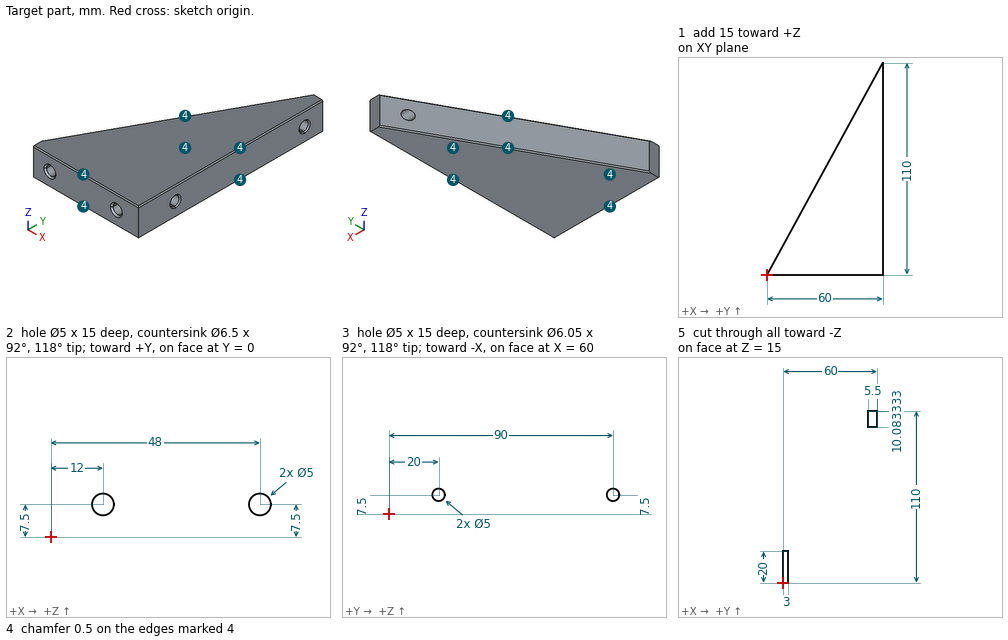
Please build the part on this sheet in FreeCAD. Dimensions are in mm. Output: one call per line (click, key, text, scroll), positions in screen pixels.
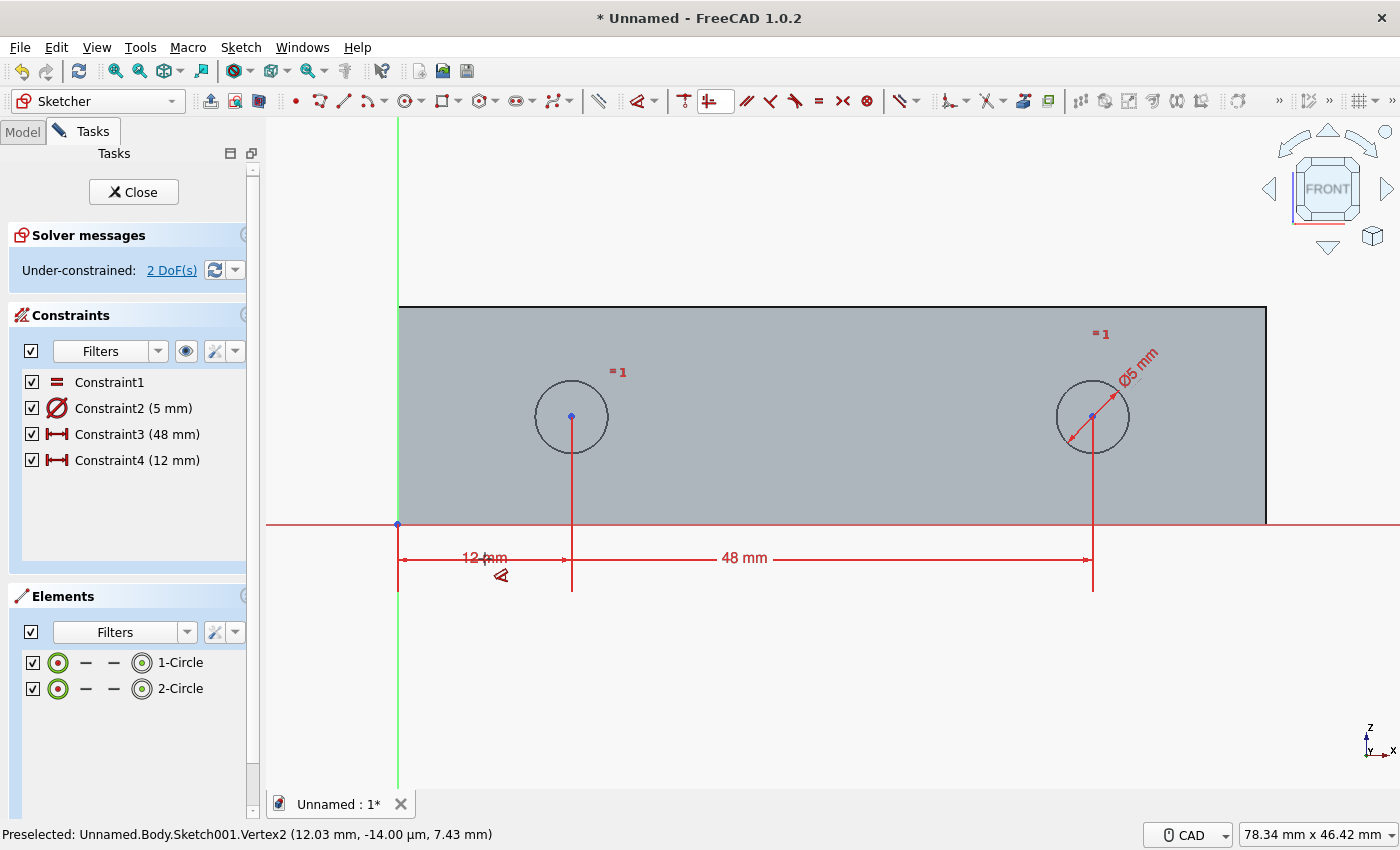
click(1093, 417)
click(364, 471)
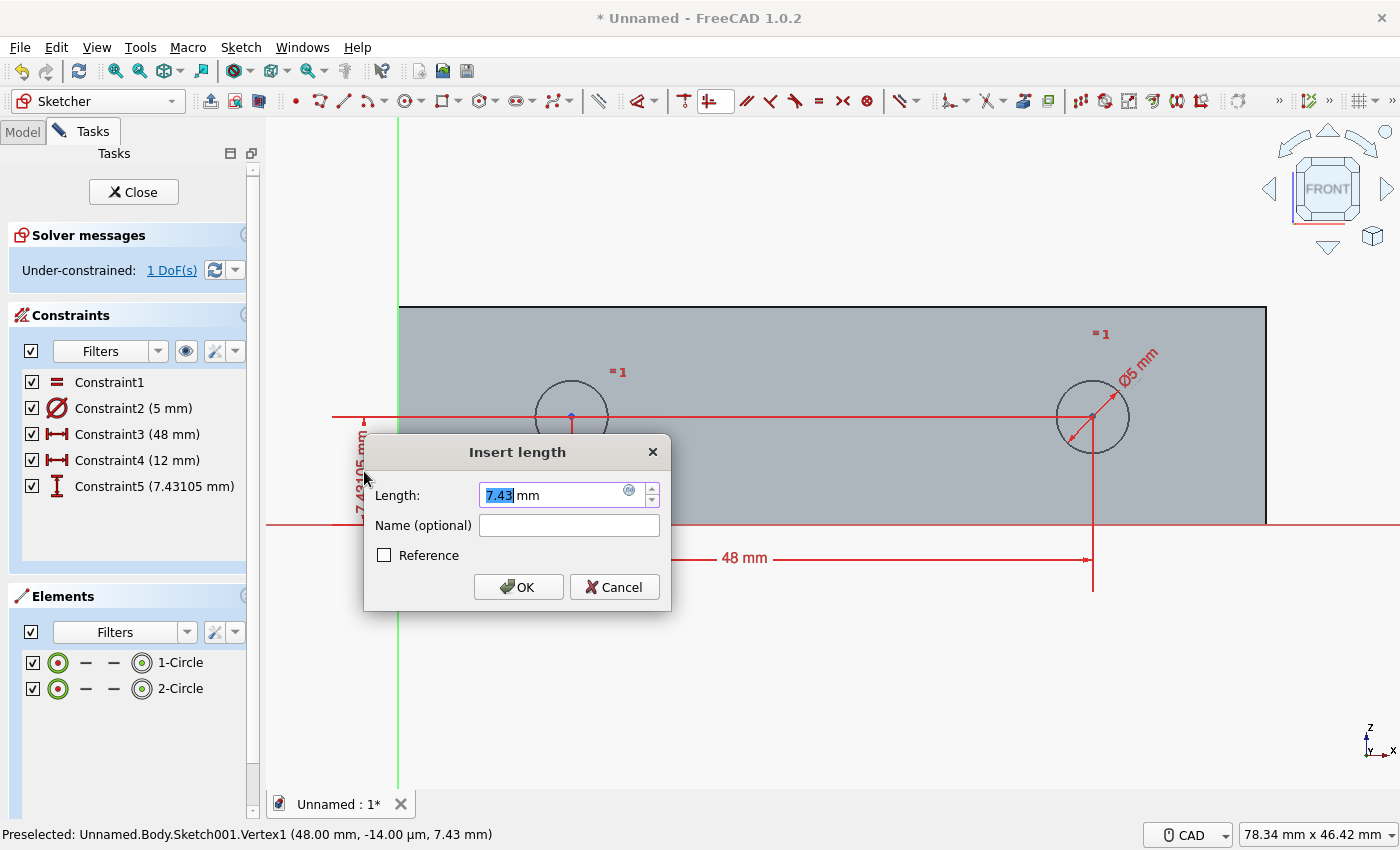
text(7.5)
key(Return)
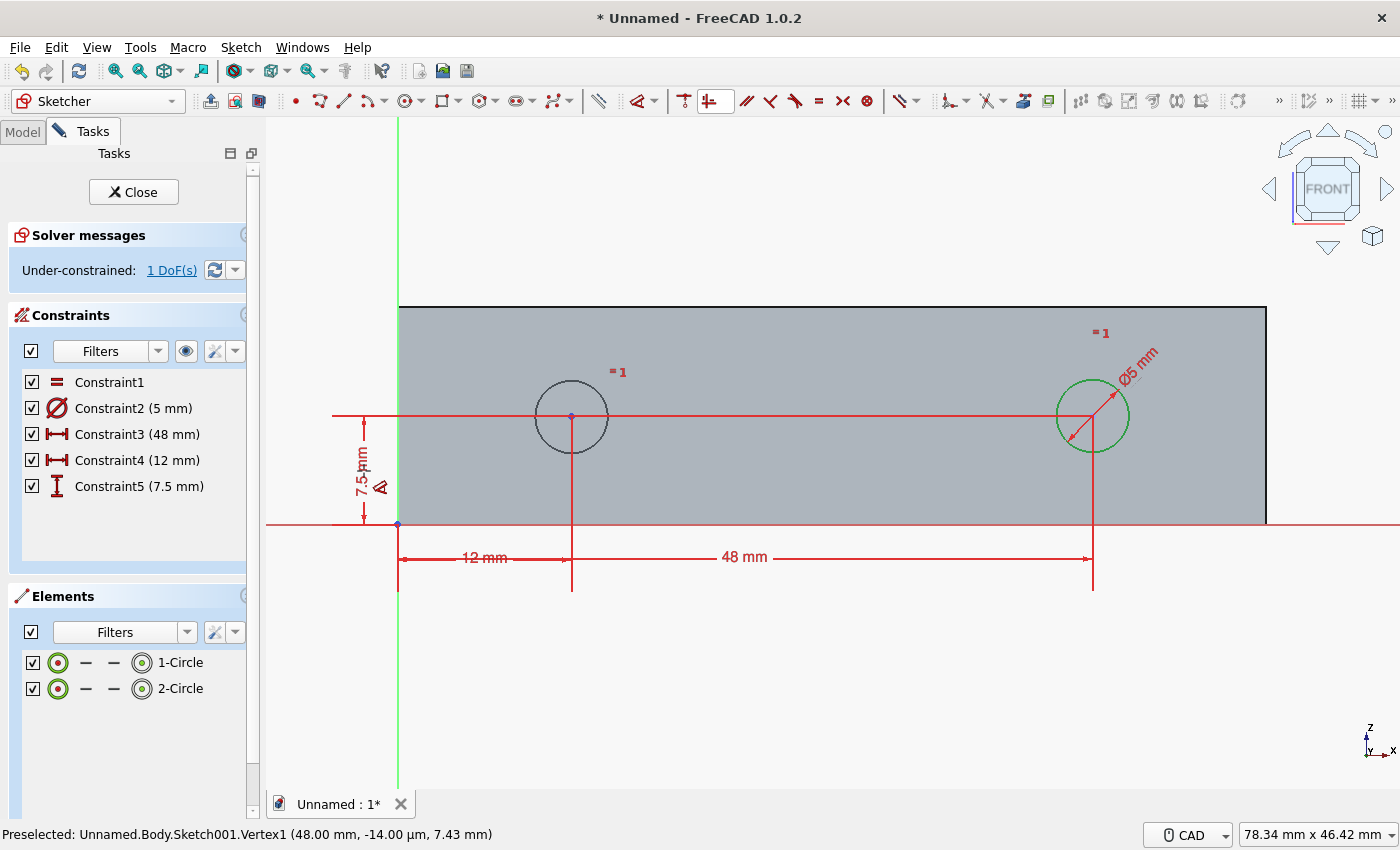
click(572, 417)
click(364, 446)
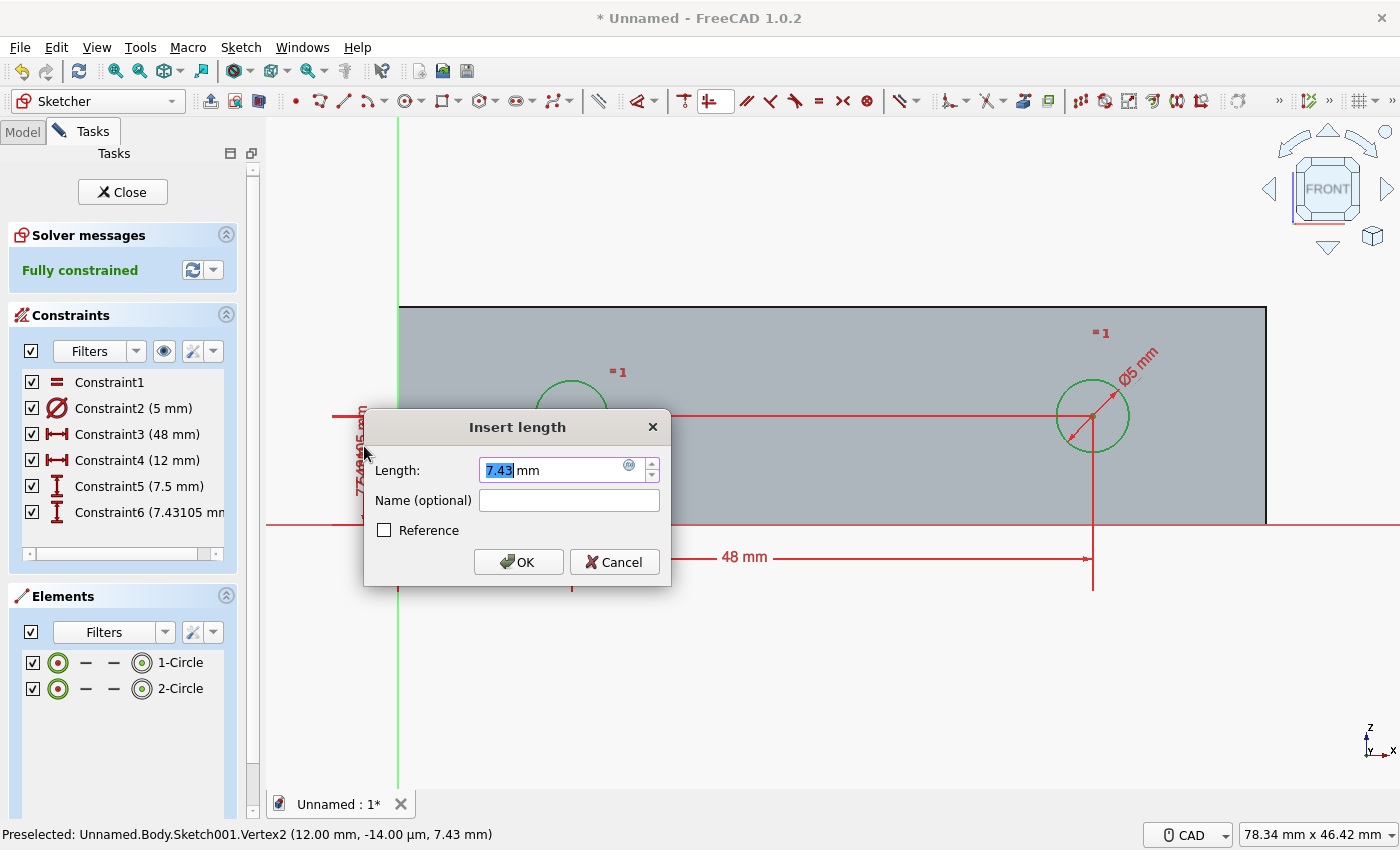
text(7.5)
key(Return)
key(Escape)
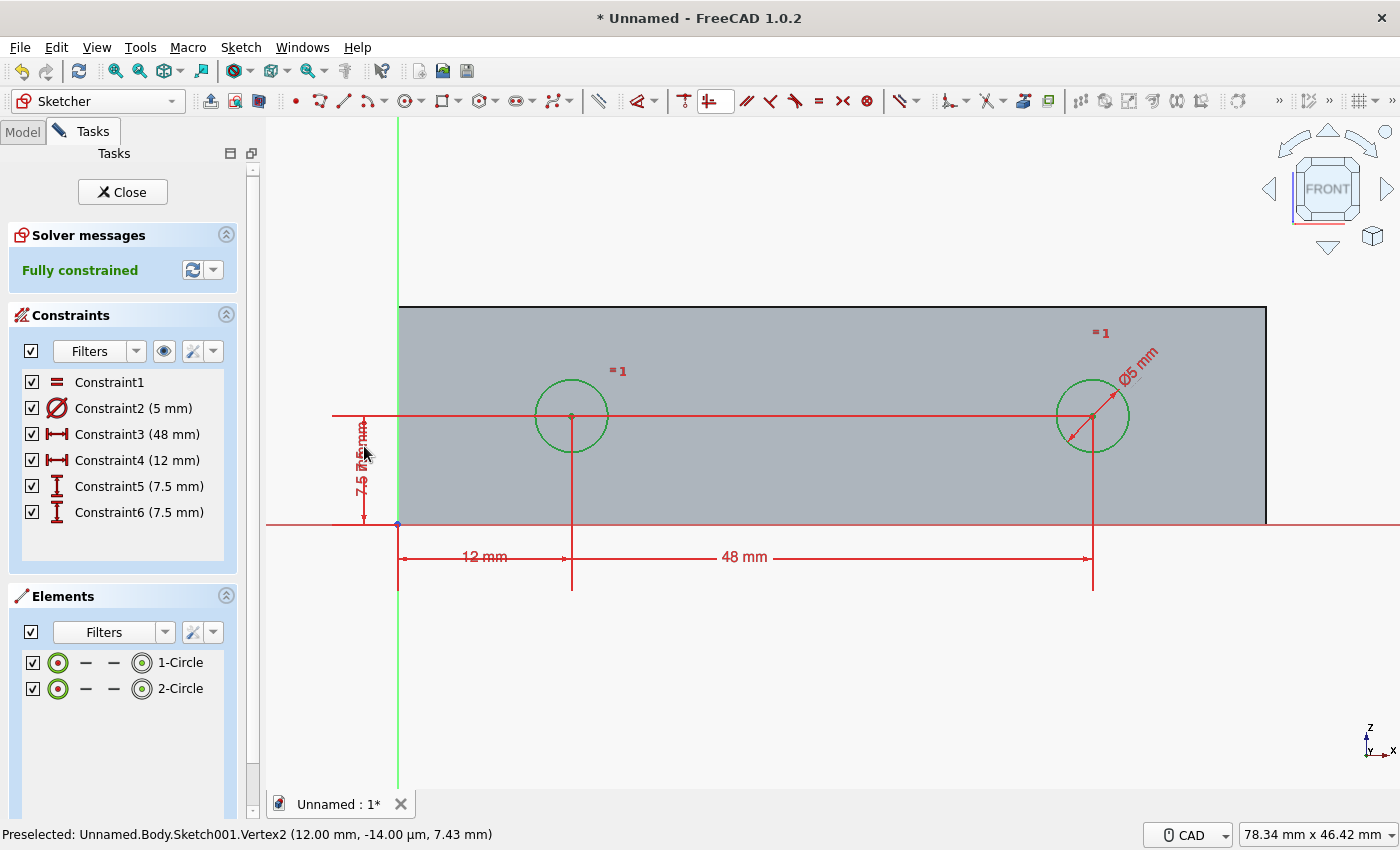
click(123, 192)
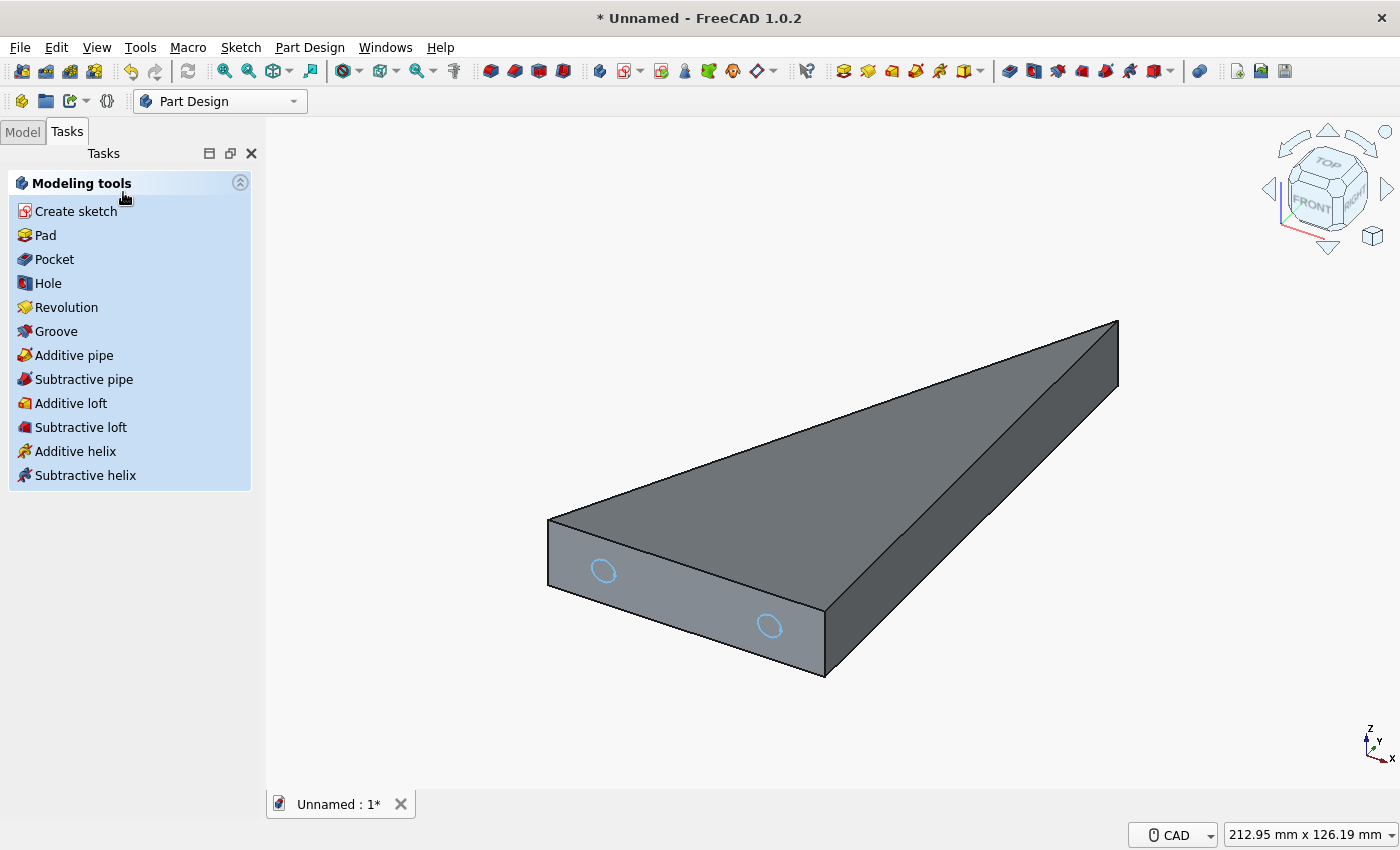
click(1034, 72)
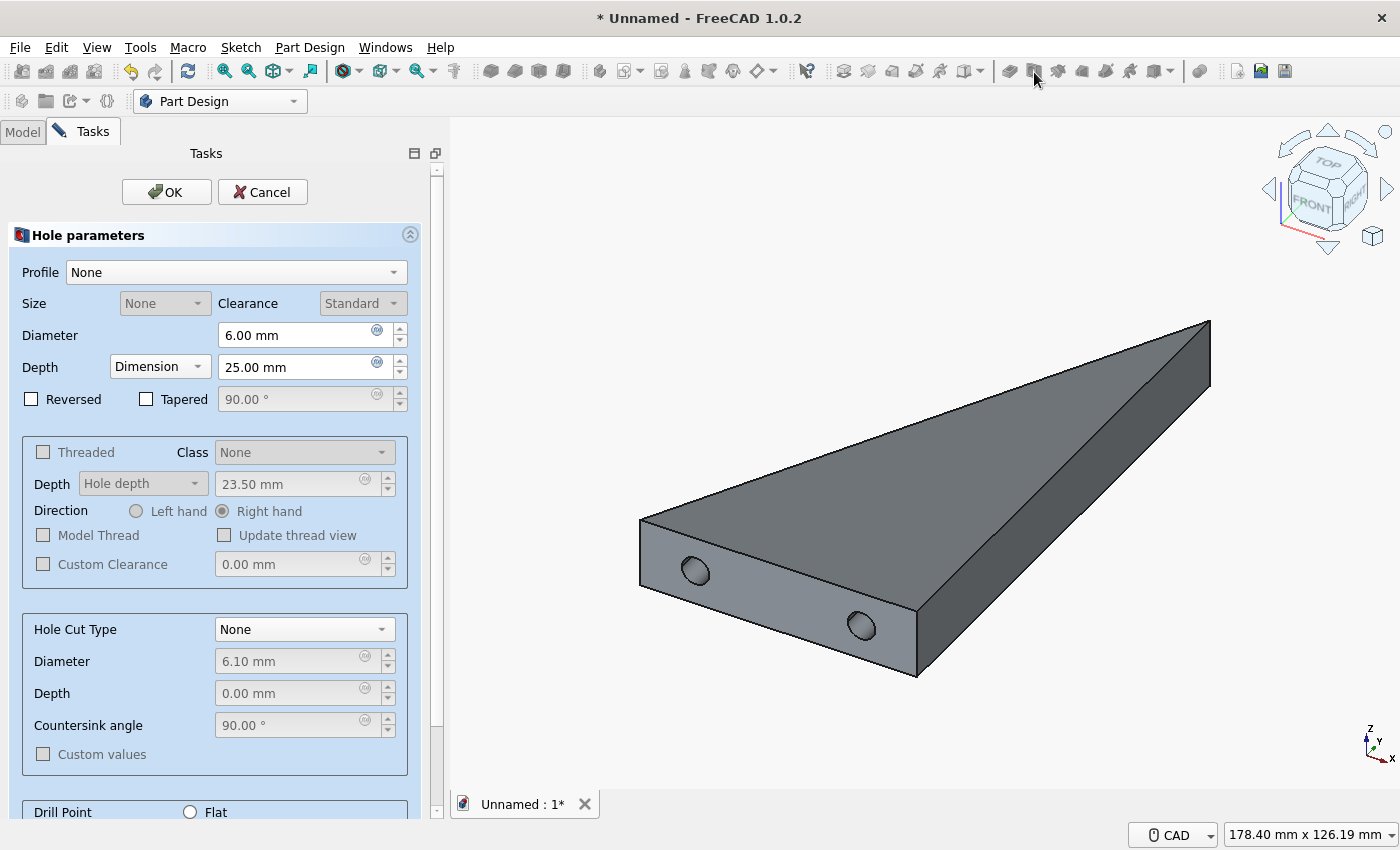
triple_click(305, 335)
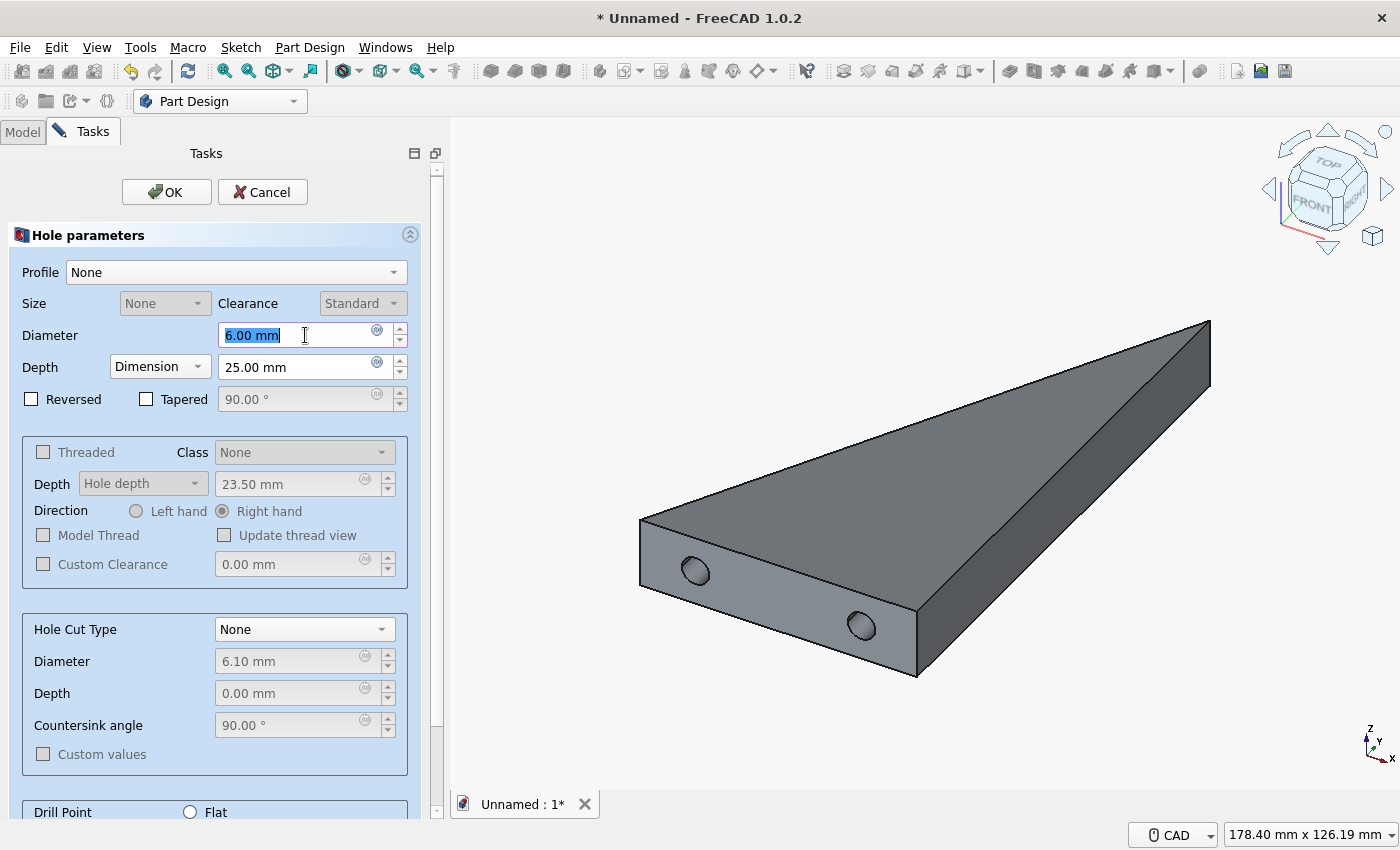
text(5)
key(Tab)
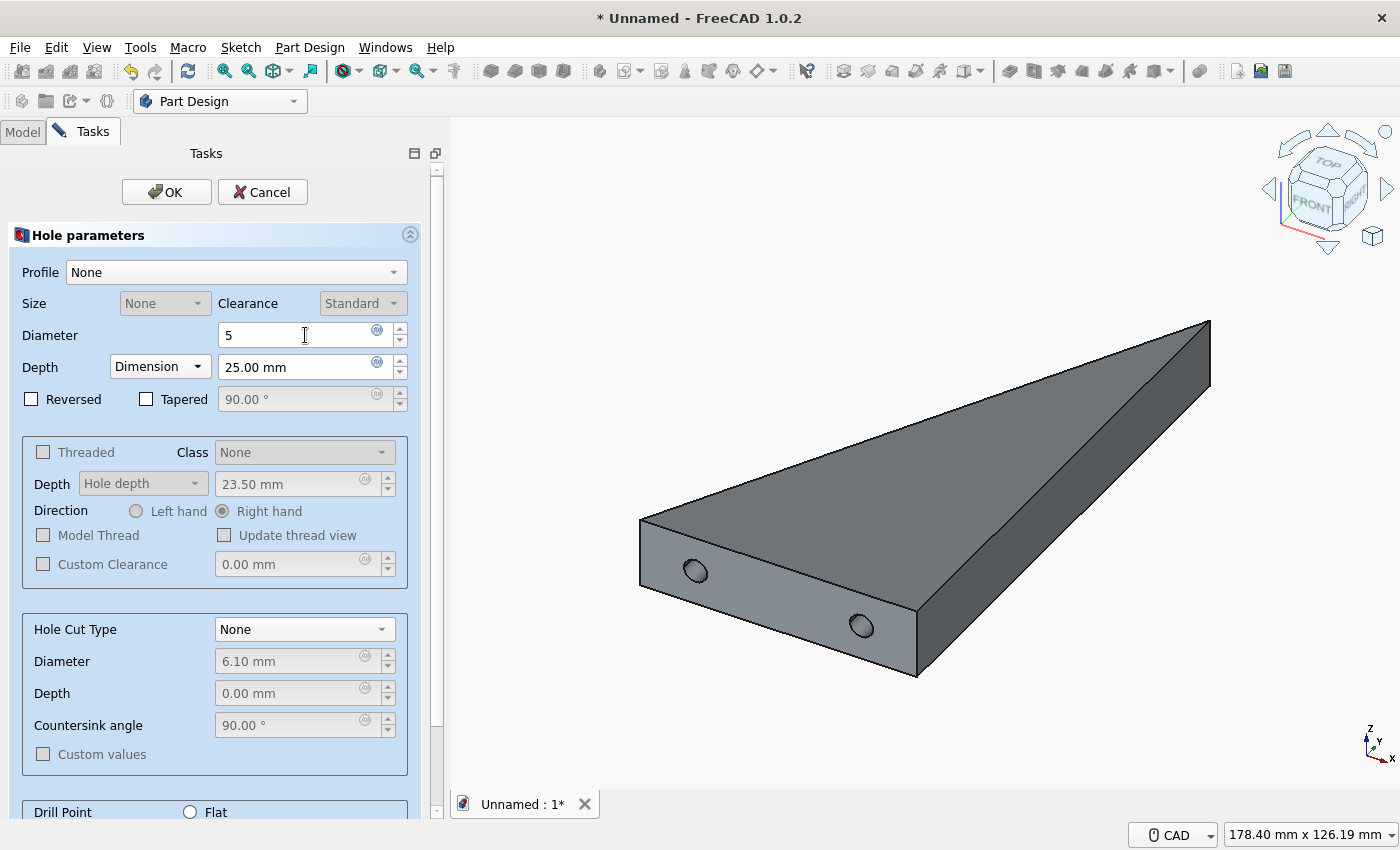
triple_click(305, 367)